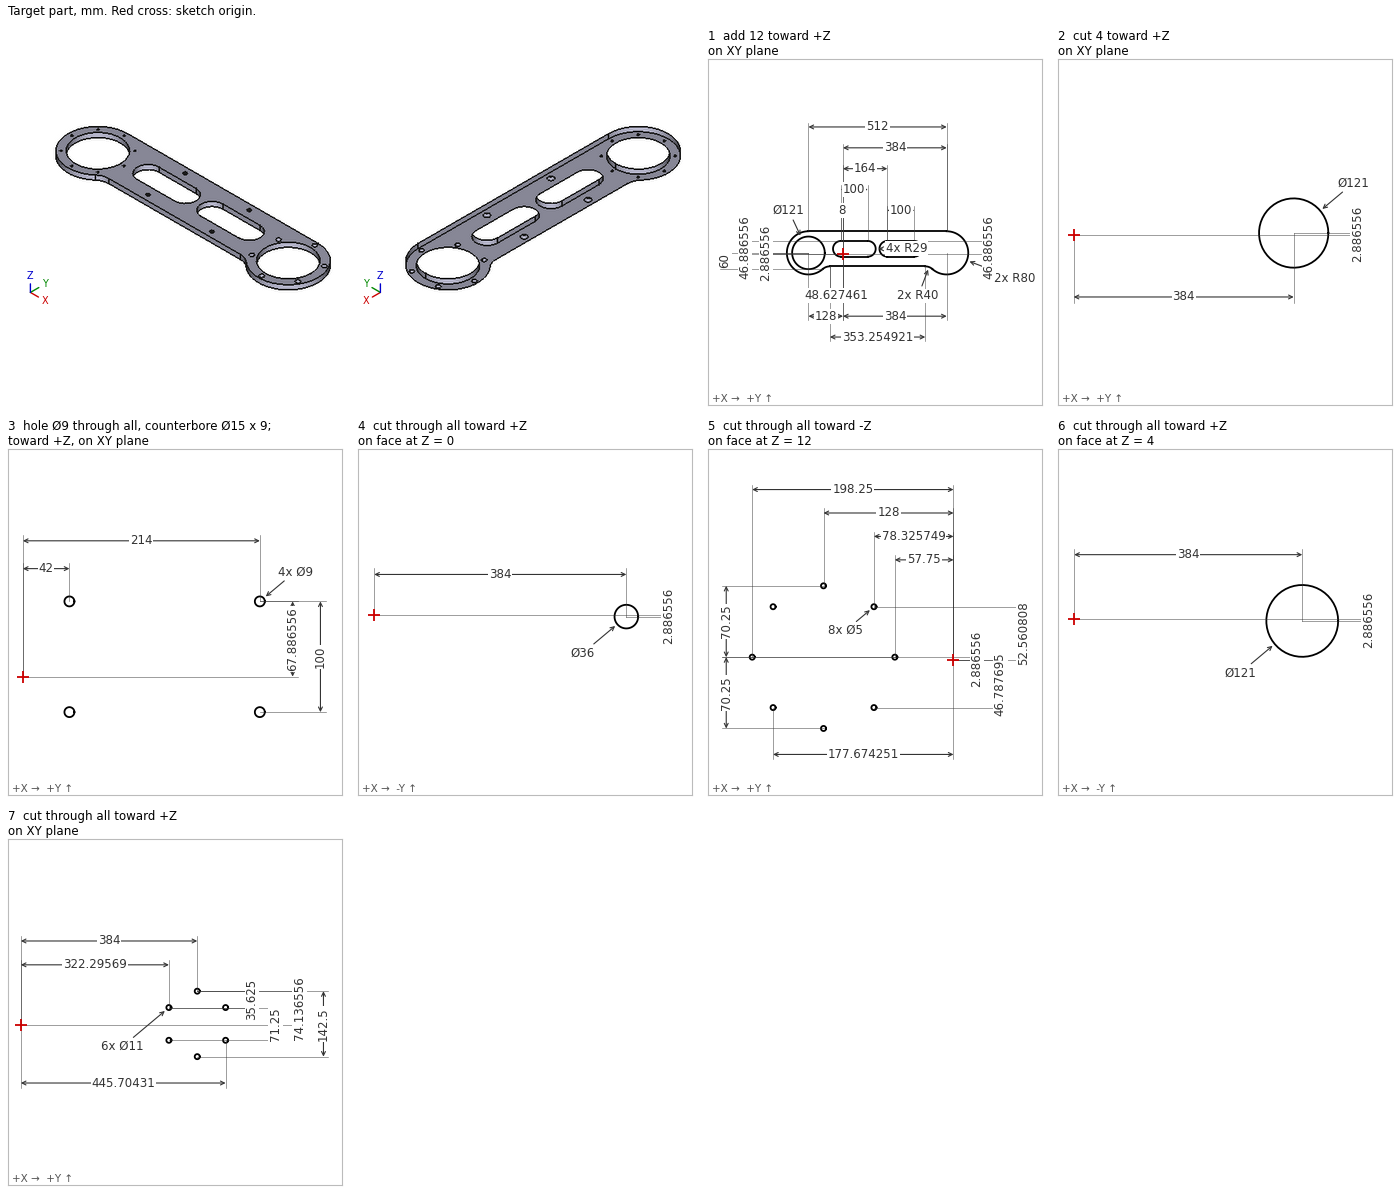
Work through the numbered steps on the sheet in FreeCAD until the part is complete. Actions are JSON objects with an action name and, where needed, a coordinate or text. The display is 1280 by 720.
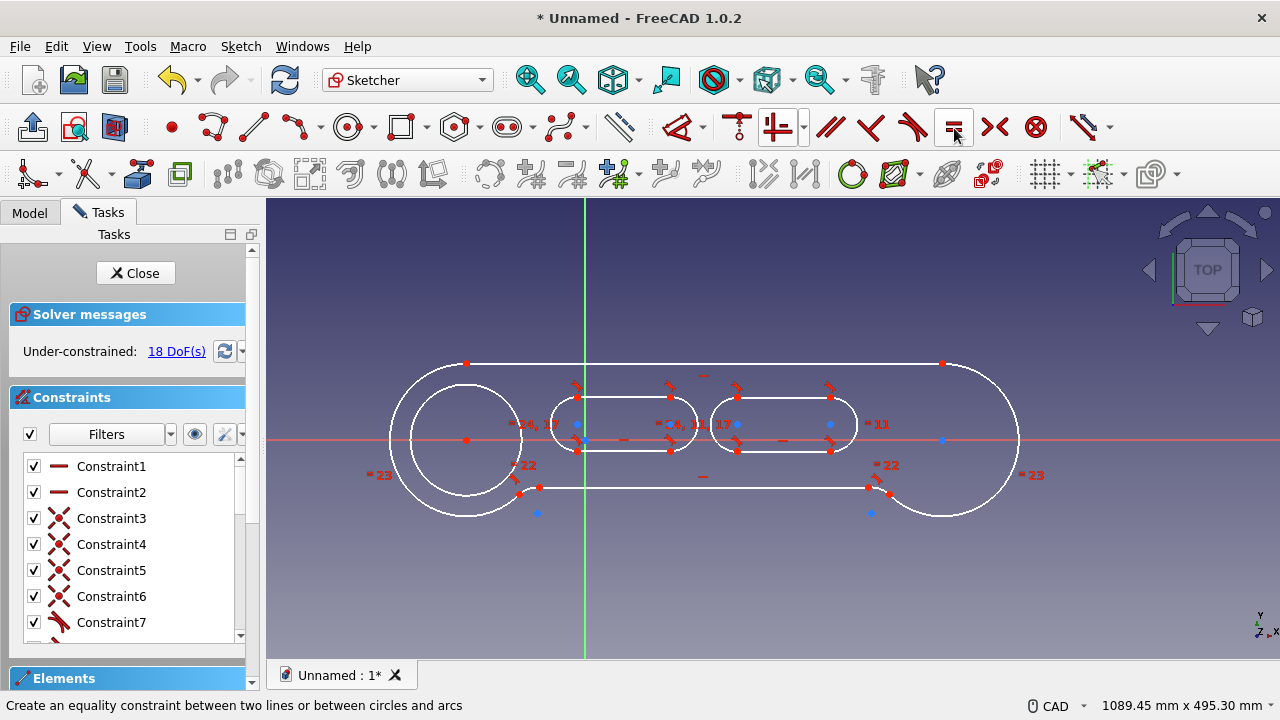
{"action": "left_click", "coordinate": [676, 128]}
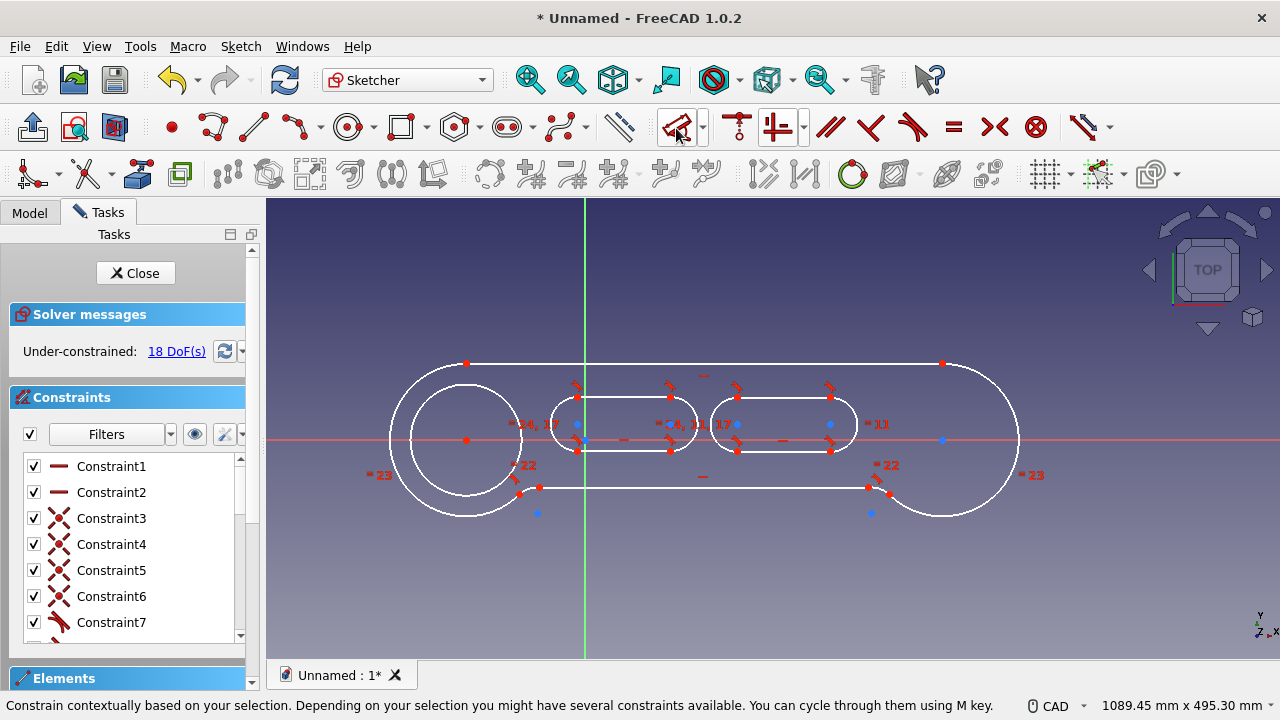
{"action": "left_click", "coordinate": [396, 410]}
{"action": "left_click", "coordinate": [367, 397]}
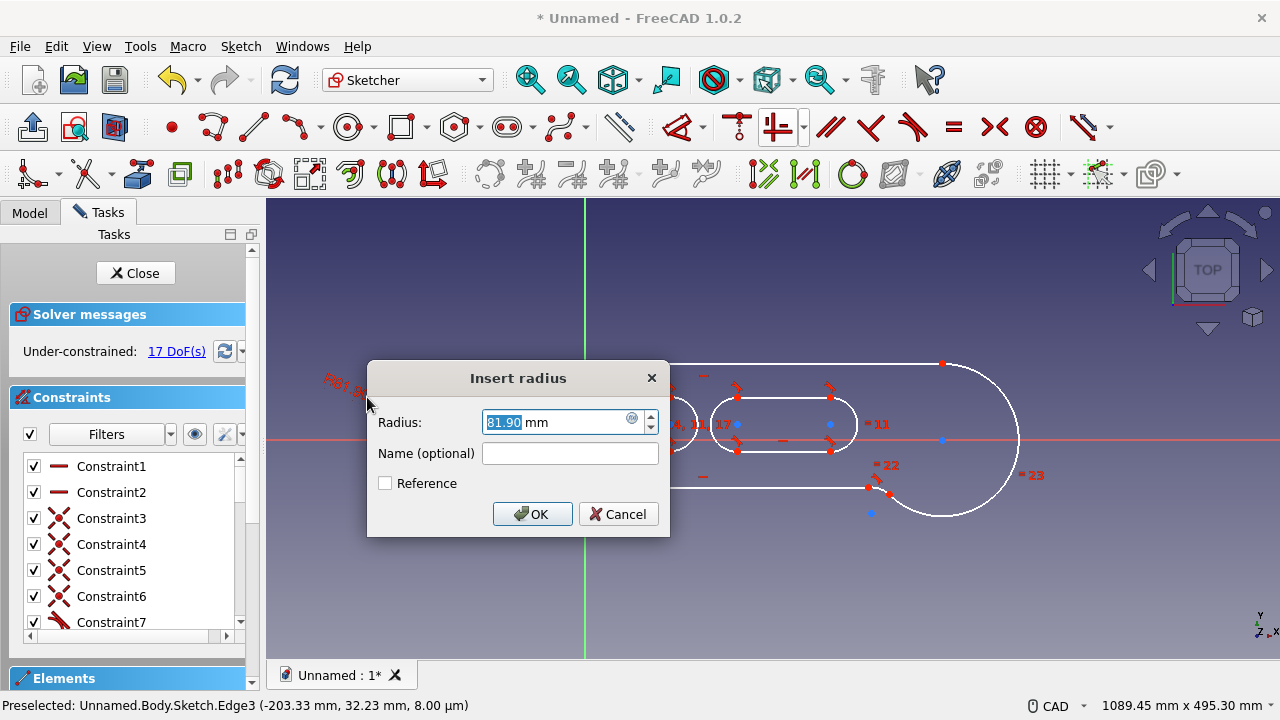
{"action": "type", "text": "80"}
{"action": "key", "text": "Return"}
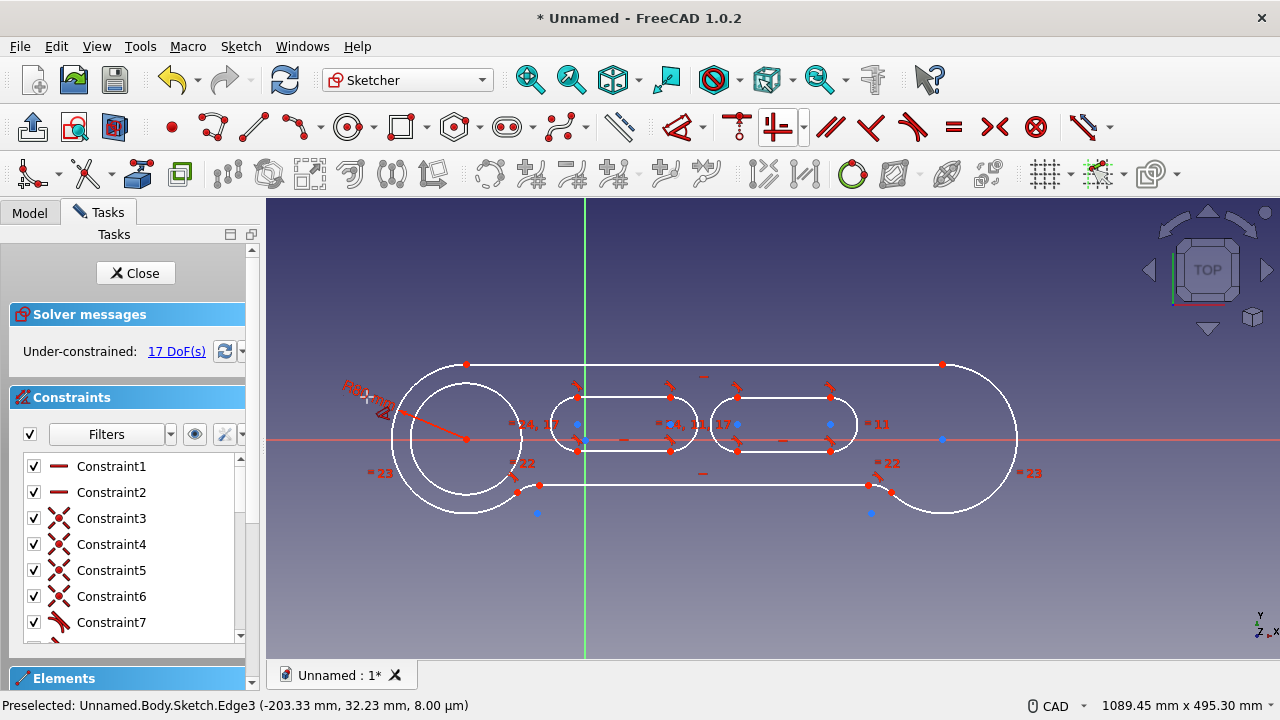
{"action": "left_click", "coordinate": [528, 487]}
{"action": "left_click", "coordinate": [547, 454]}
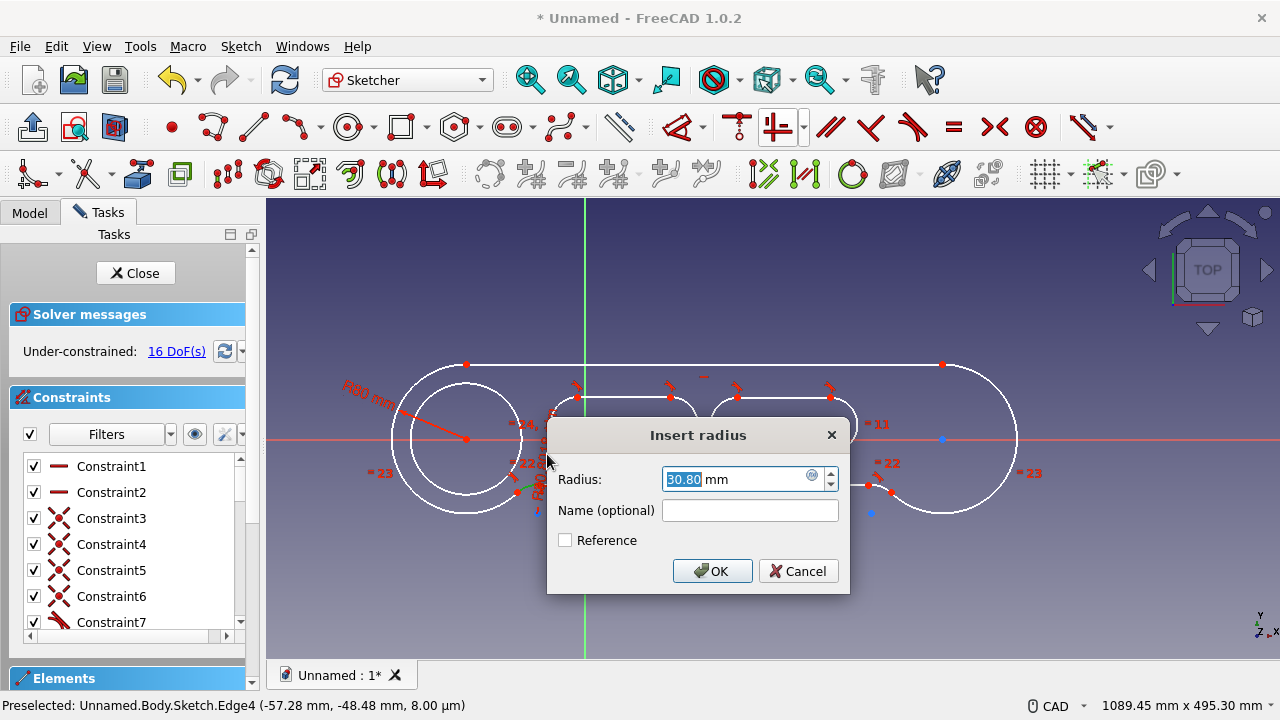
{"action": "type", "text": "40"}
{"action": "key", "text": "Return"}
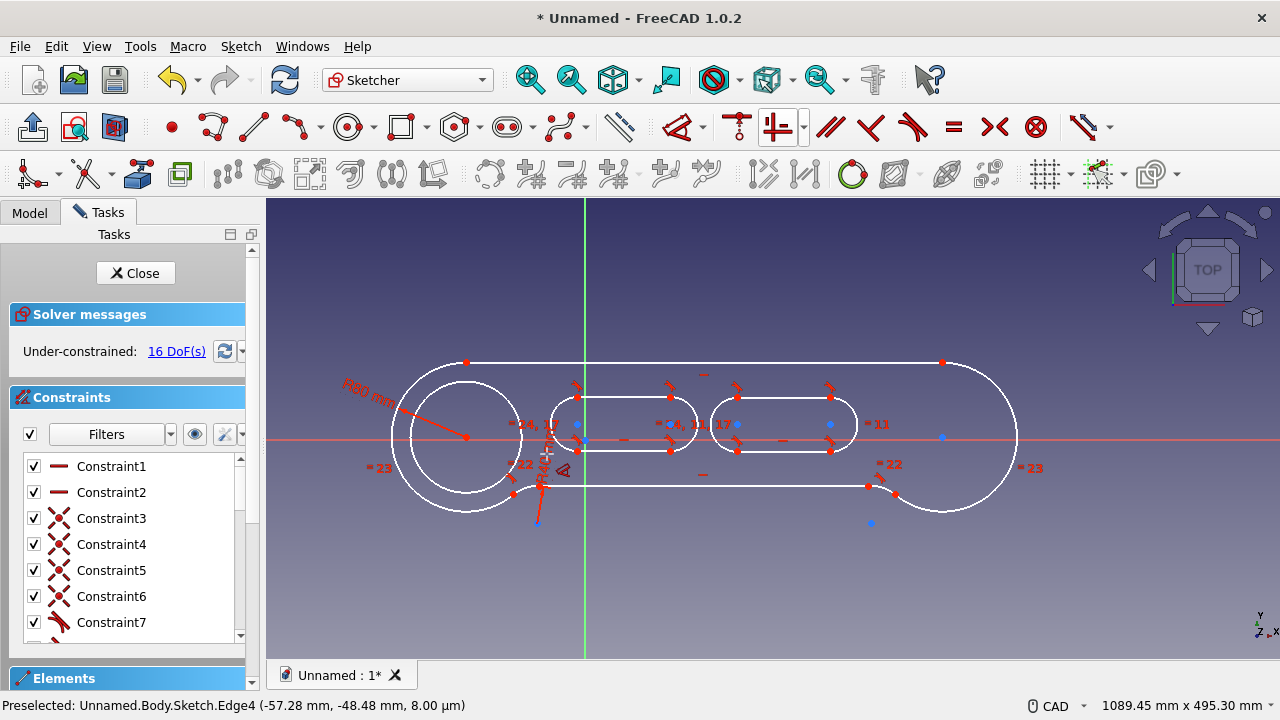
{"action": "scroll", "coordinate": [716, 409], "scroll_direction": "up", "scroll_amount": 2}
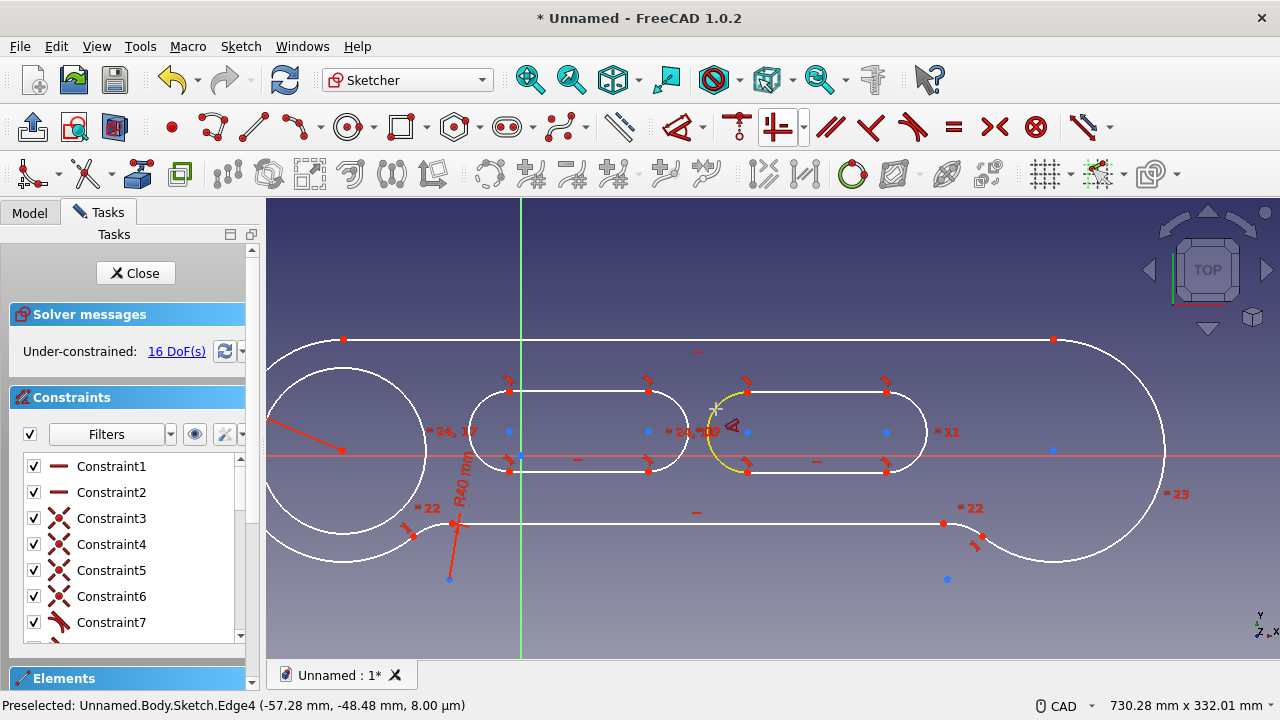
{"action": "left_click", "coordinate": [715, 409]}
{"action": "left_click", "coordinate": [689, 390]}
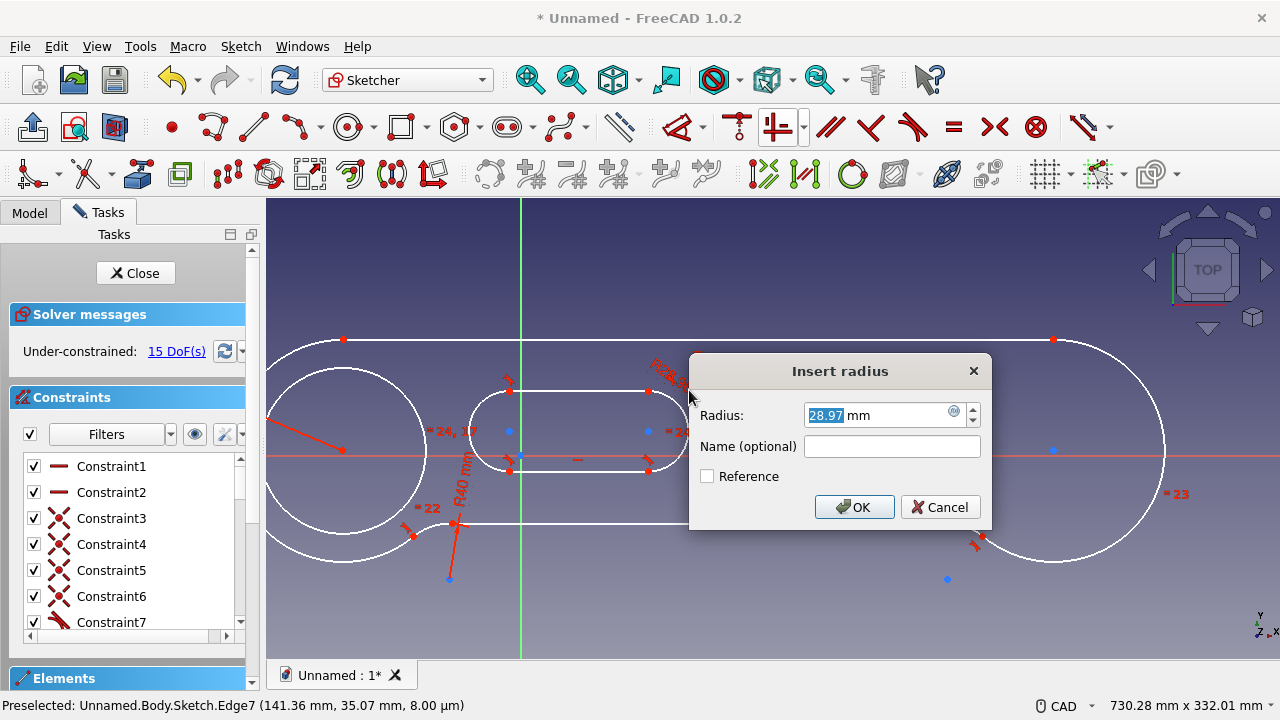
{"action": "type", "text": "29"}
{"action": "key", "text": "Return"}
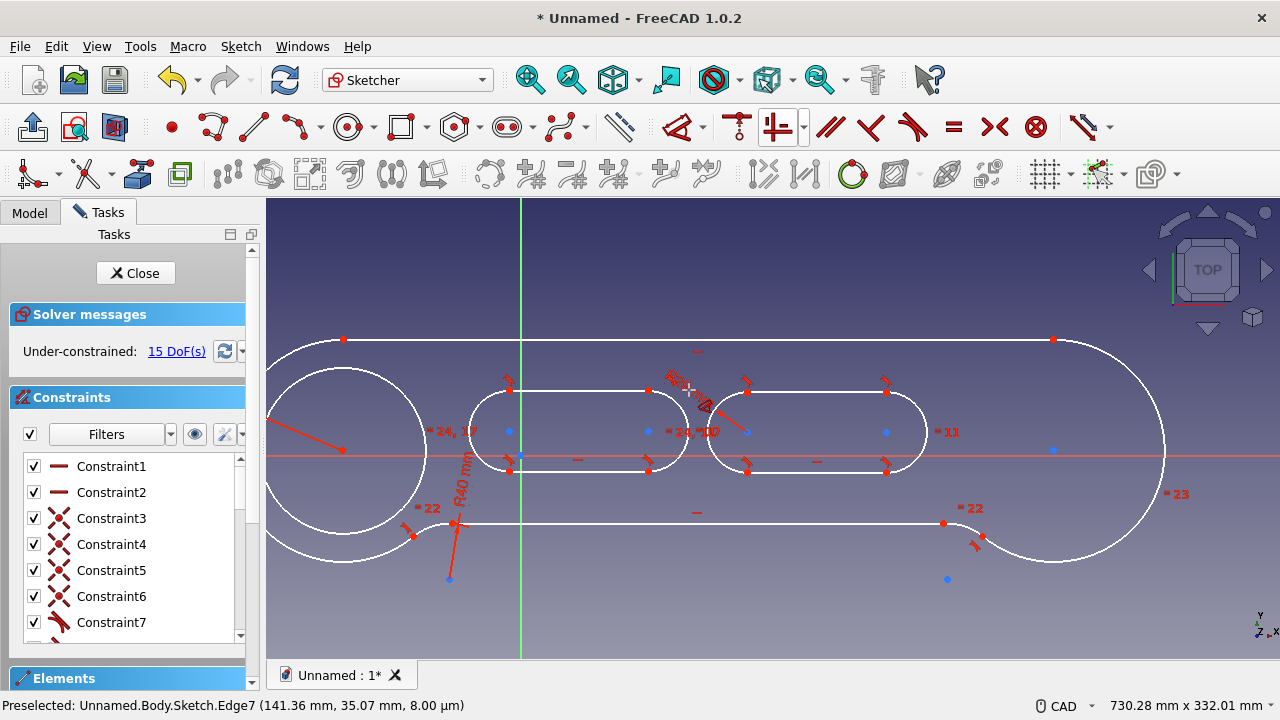
{"action": "left_click", "coordinate": [401, 392]}
{"action": "left_click", "coordinate": [423, 369]}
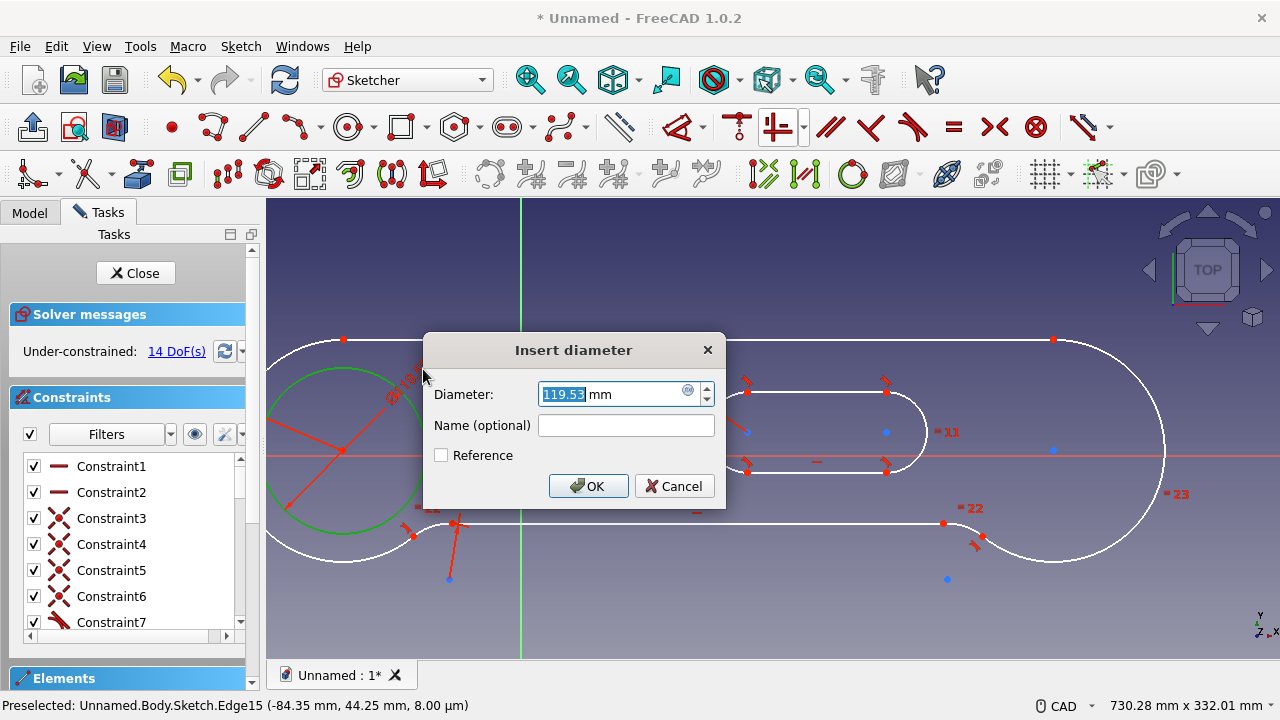
{"action": "type", "text": "121"}
{"action": "key", "text": "Return"}